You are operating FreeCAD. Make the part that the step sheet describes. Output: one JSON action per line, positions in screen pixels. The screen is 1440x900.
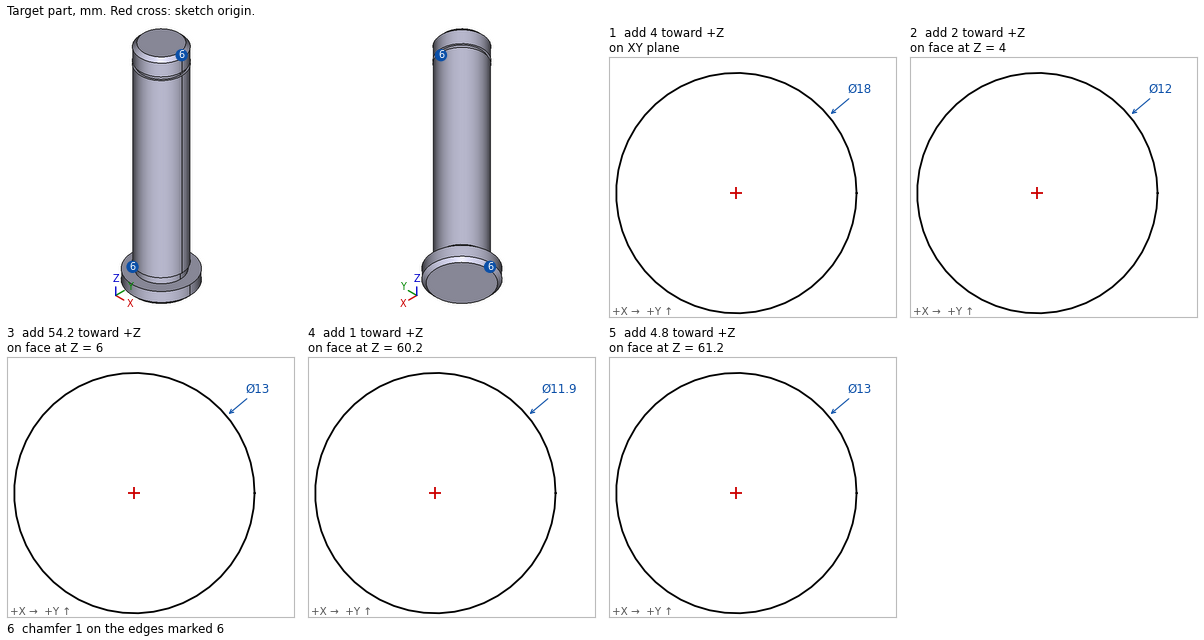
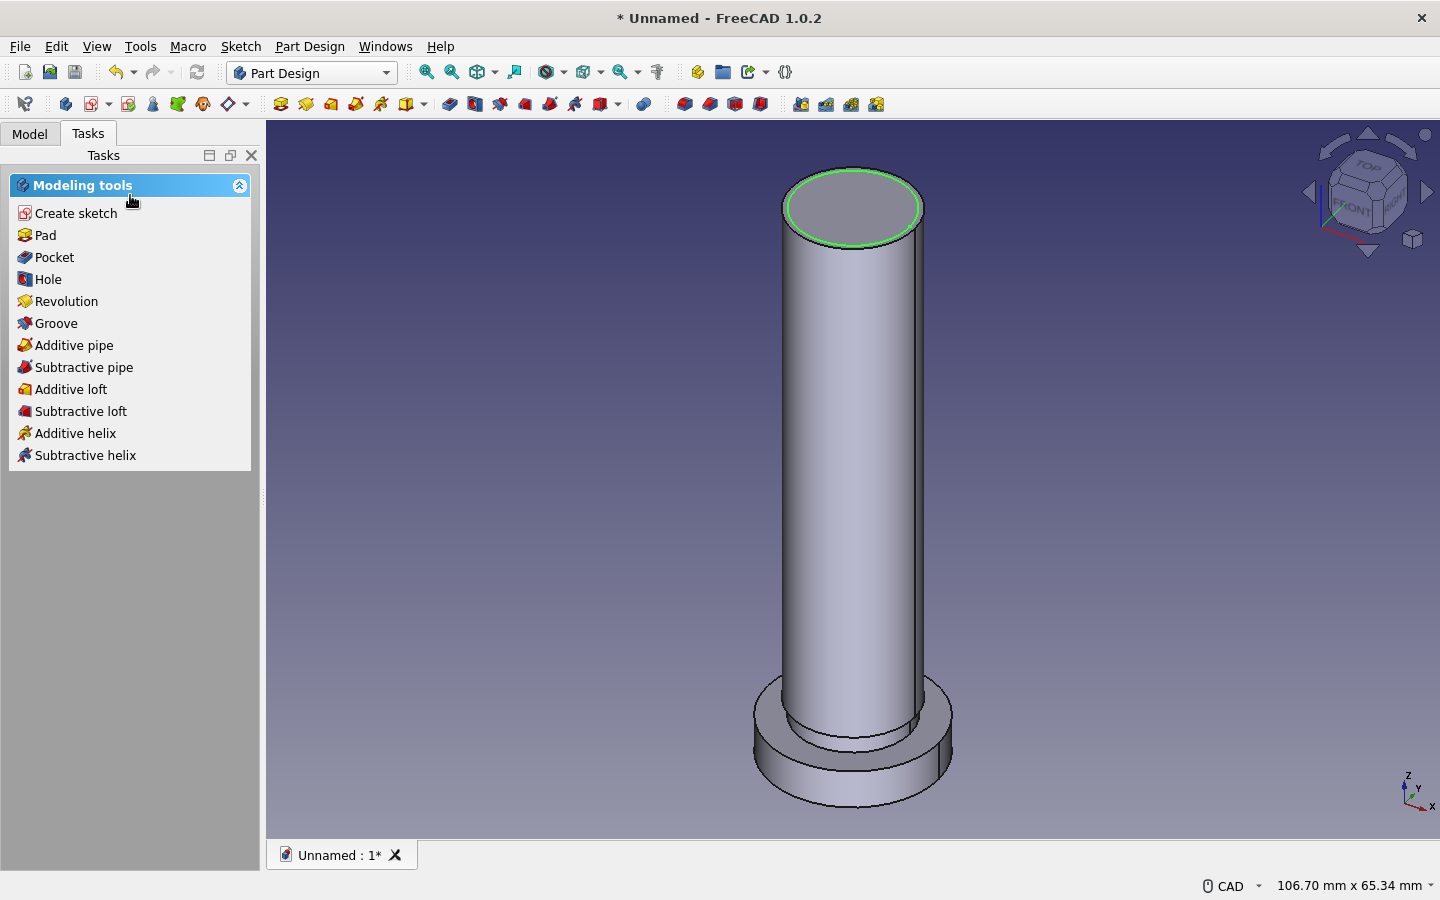
{"action": "left_click", "coordinate": [281, 104]}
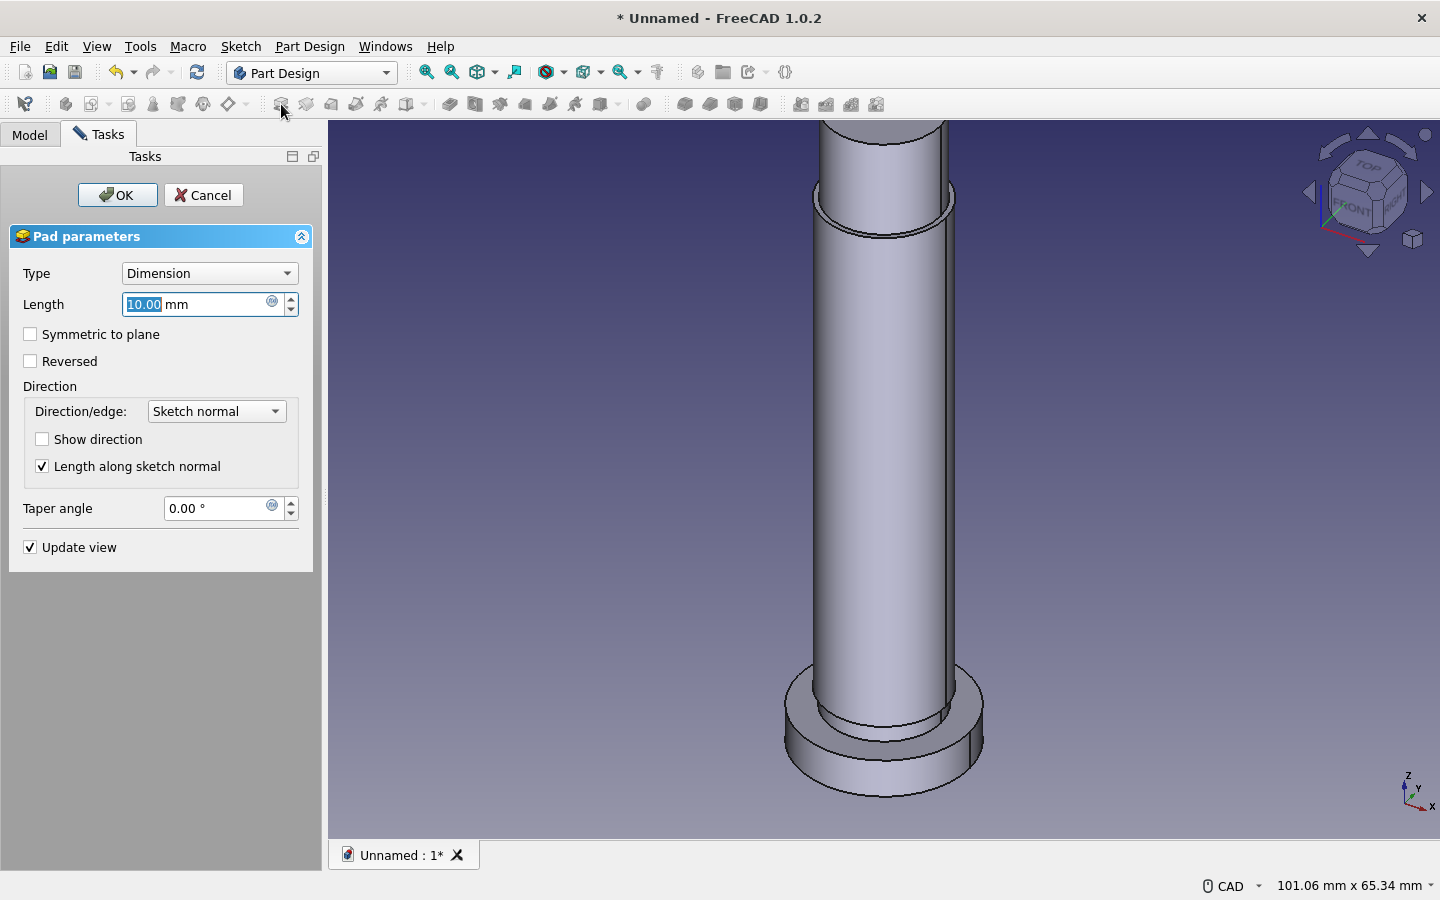
{"action": "type", "text": "1"}
{"action": "key", "text": "Tab"}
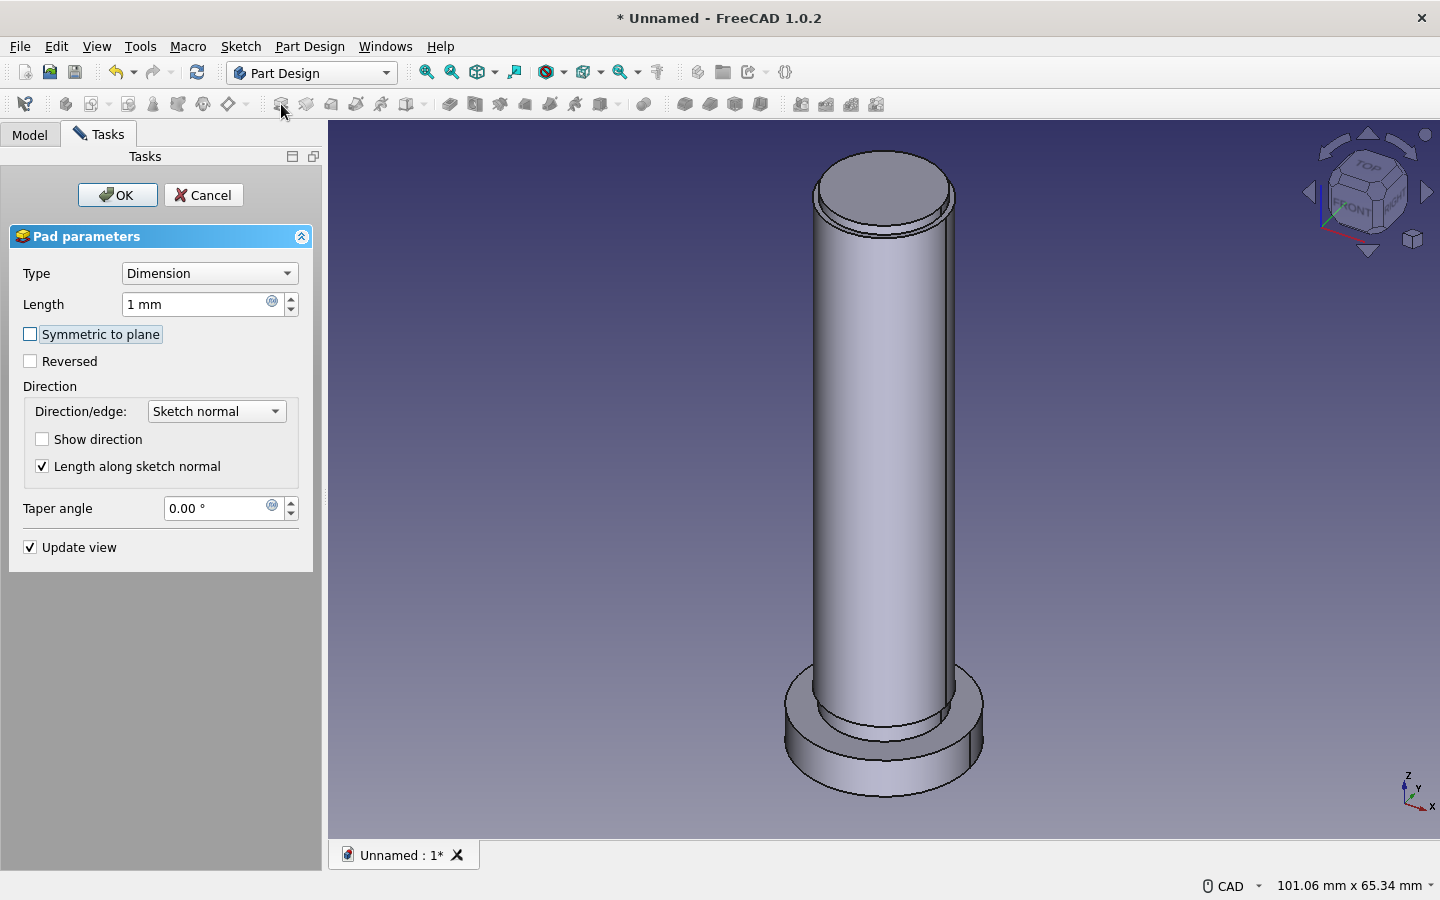
{"action": "left_click", "coordinate": [118, 195]}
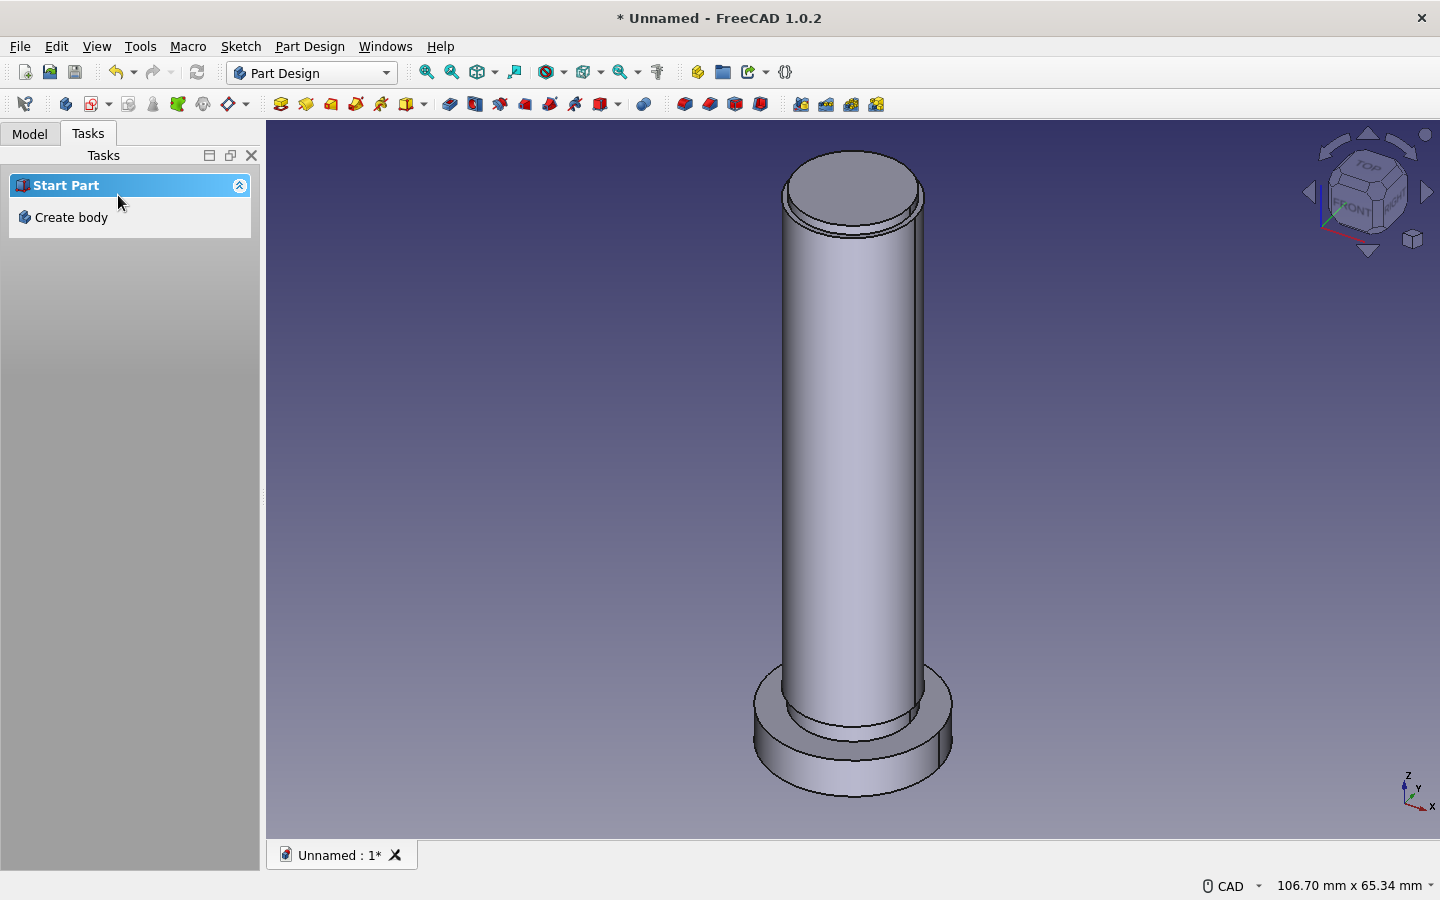
{"action": "left_click", "coordinate": [427, 72]}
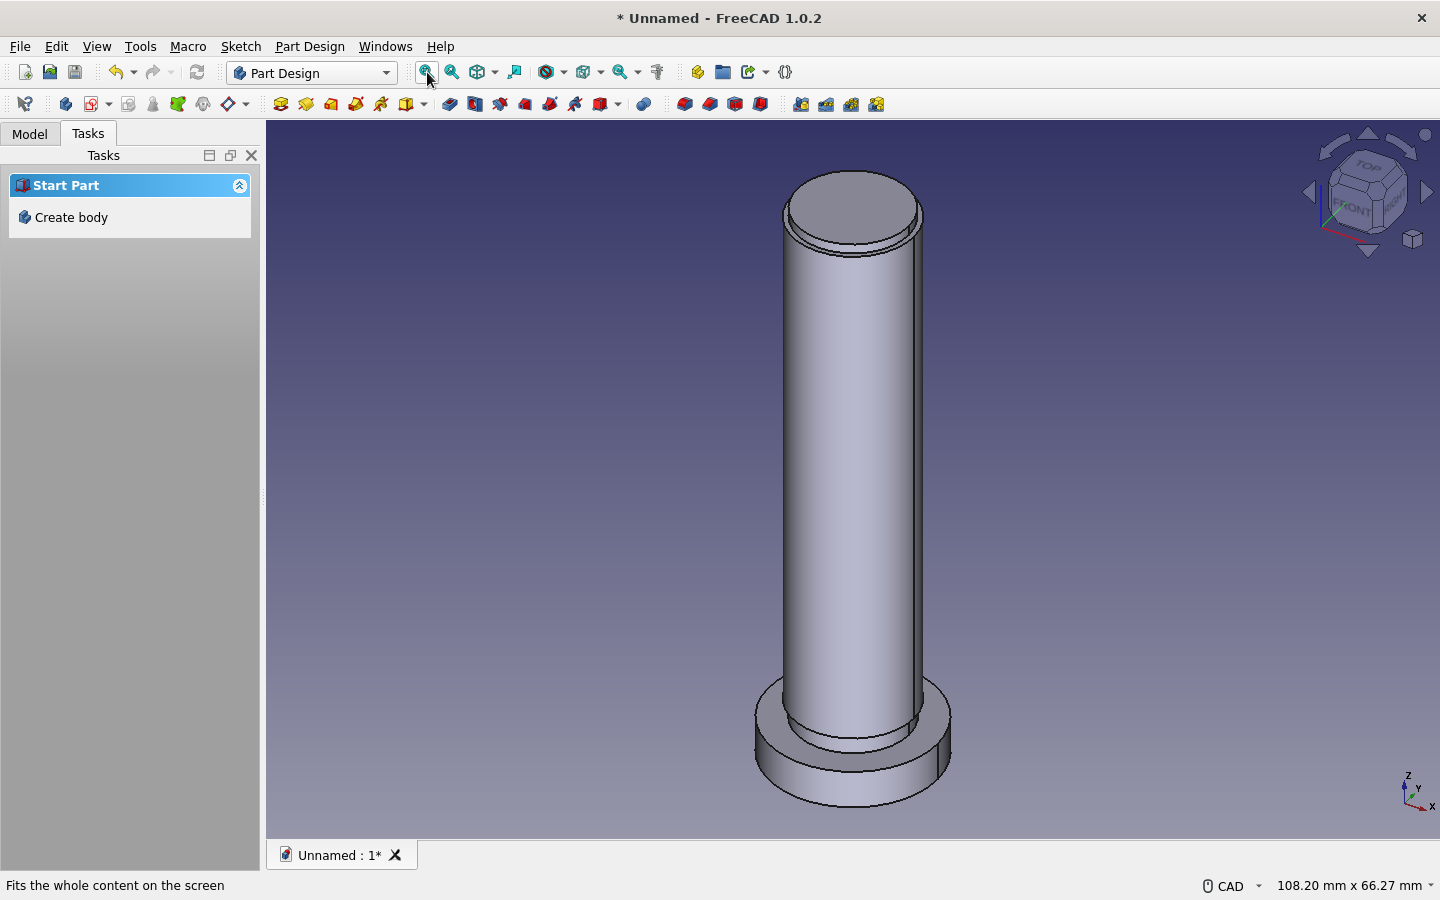
{"action": "left_click", "coordinate": [853, 207]}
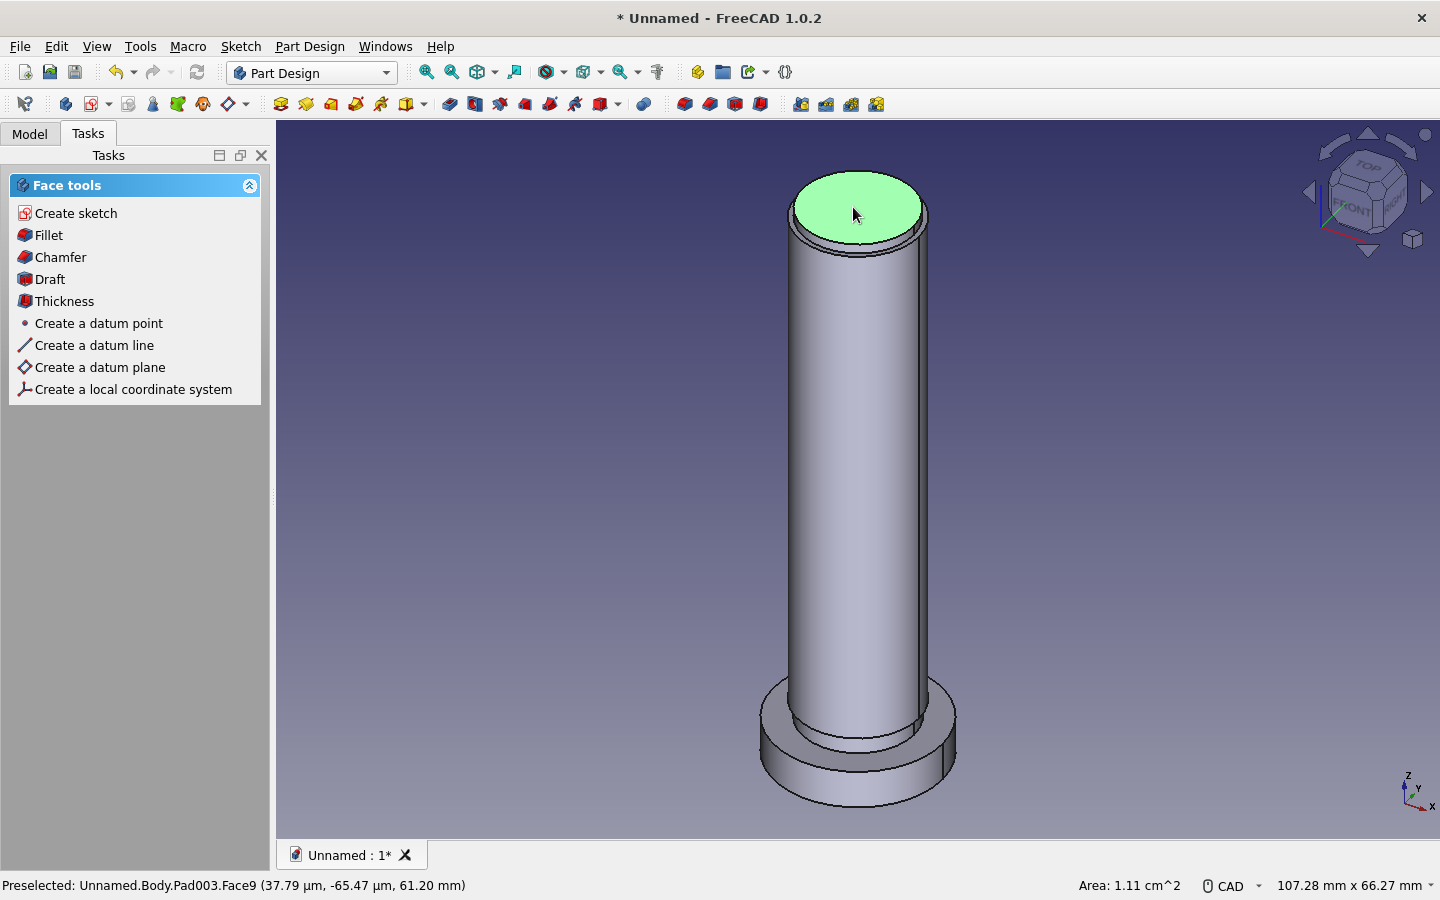
{"action": "left_click", "coordinate": [90, 104]}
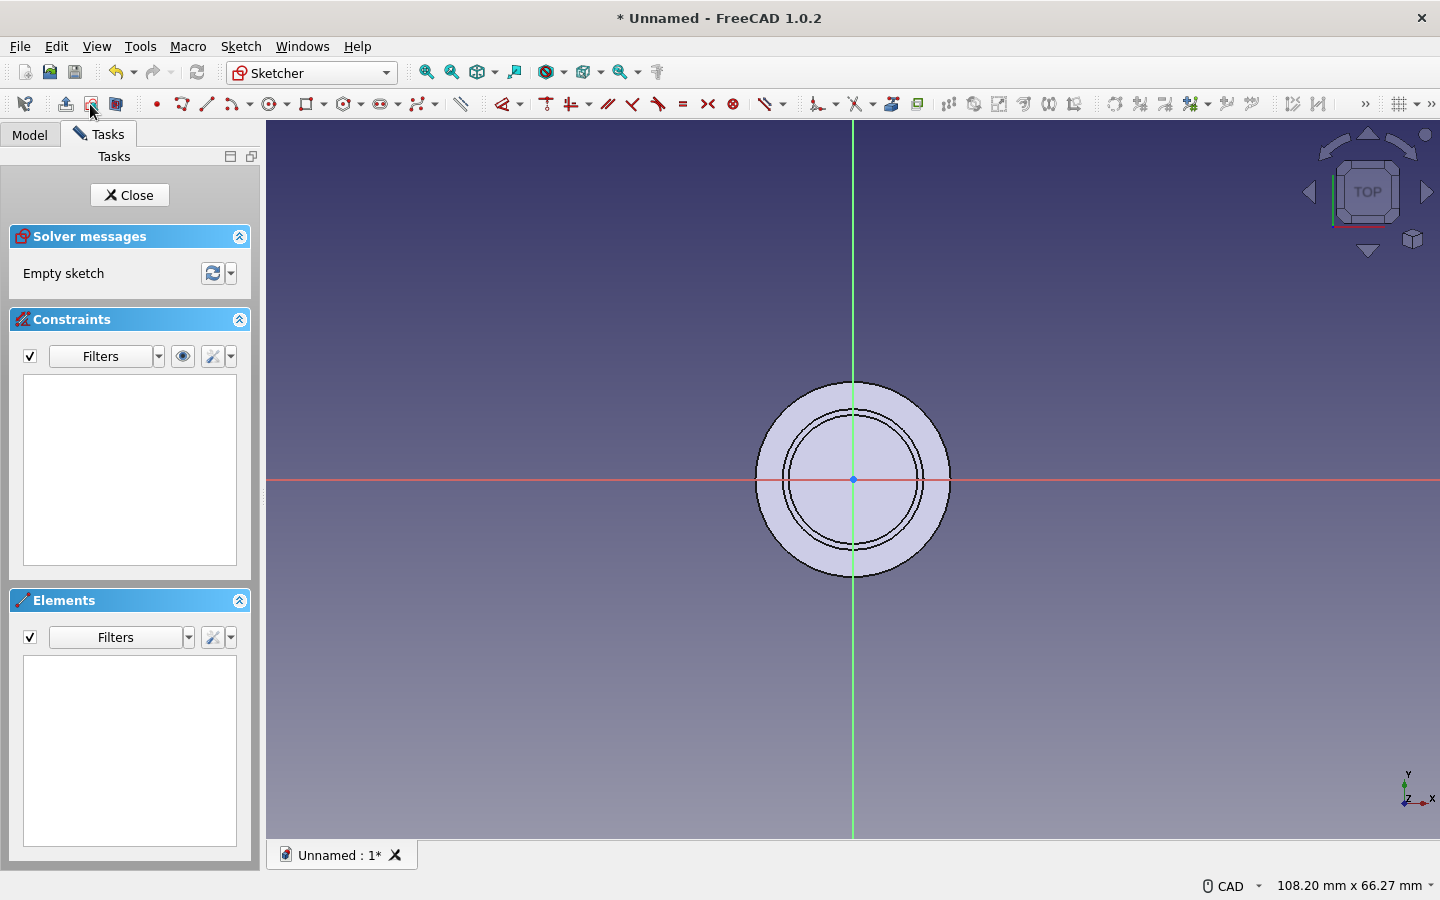
{"action": "scroll", "coordinate": [883, 480], "scroll_direction": "up", "scroll_amount": 6}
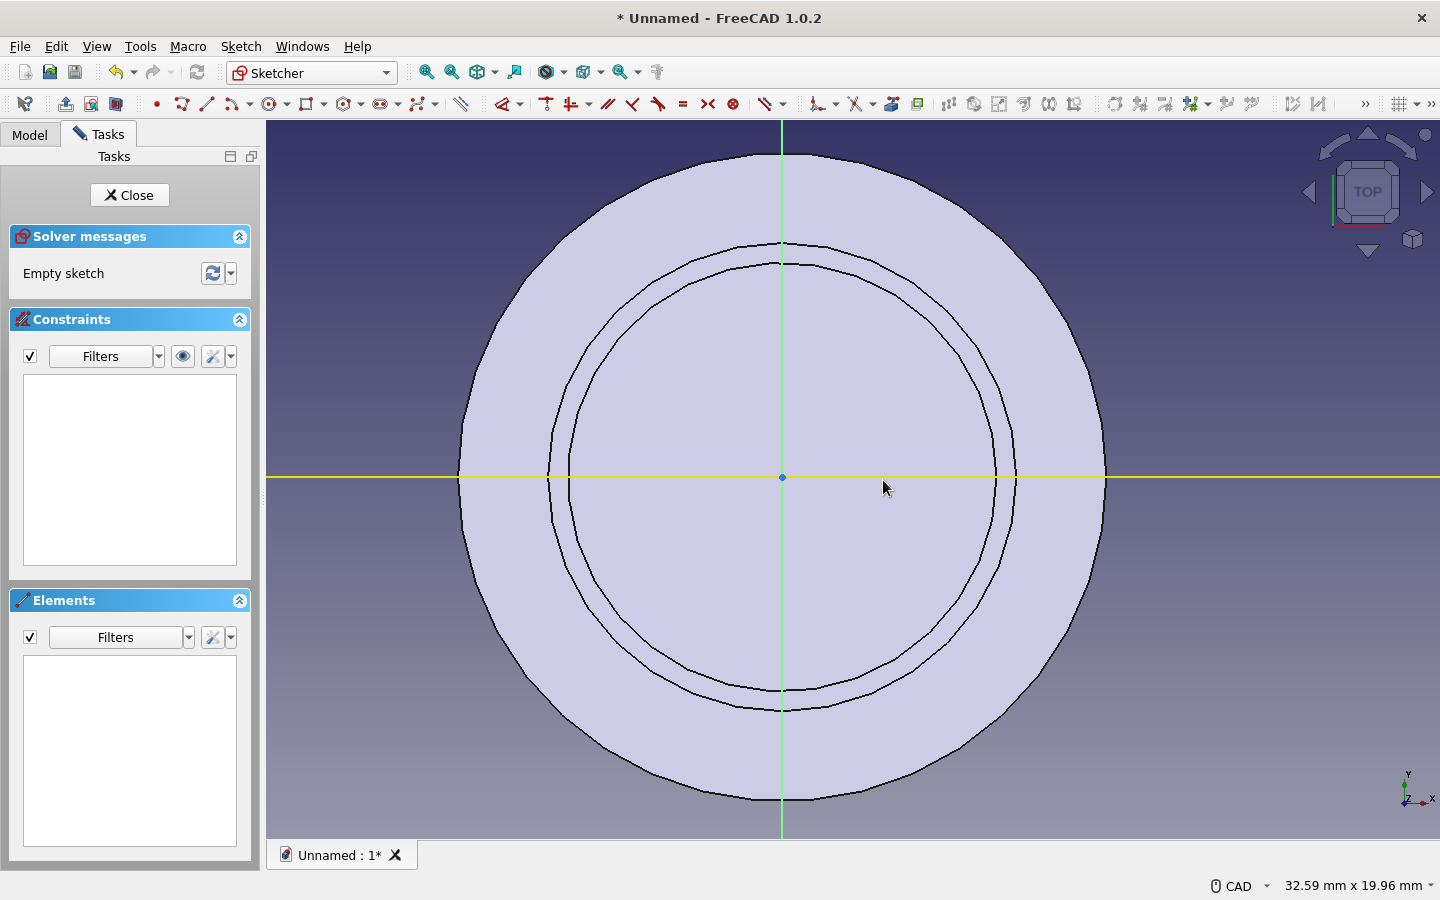
{"action": "left_click", "coordinate": [268, 104]}